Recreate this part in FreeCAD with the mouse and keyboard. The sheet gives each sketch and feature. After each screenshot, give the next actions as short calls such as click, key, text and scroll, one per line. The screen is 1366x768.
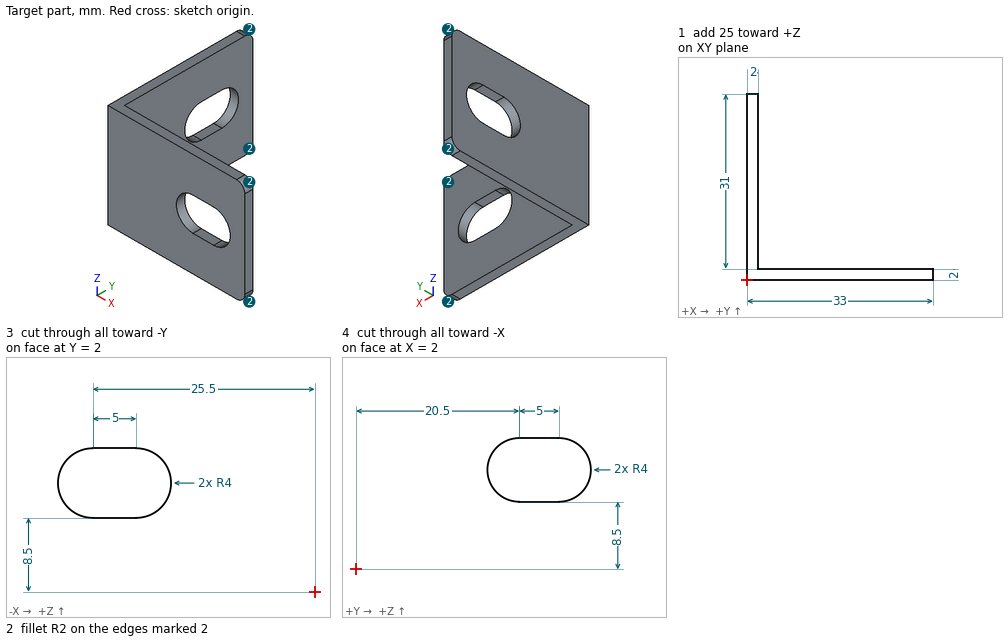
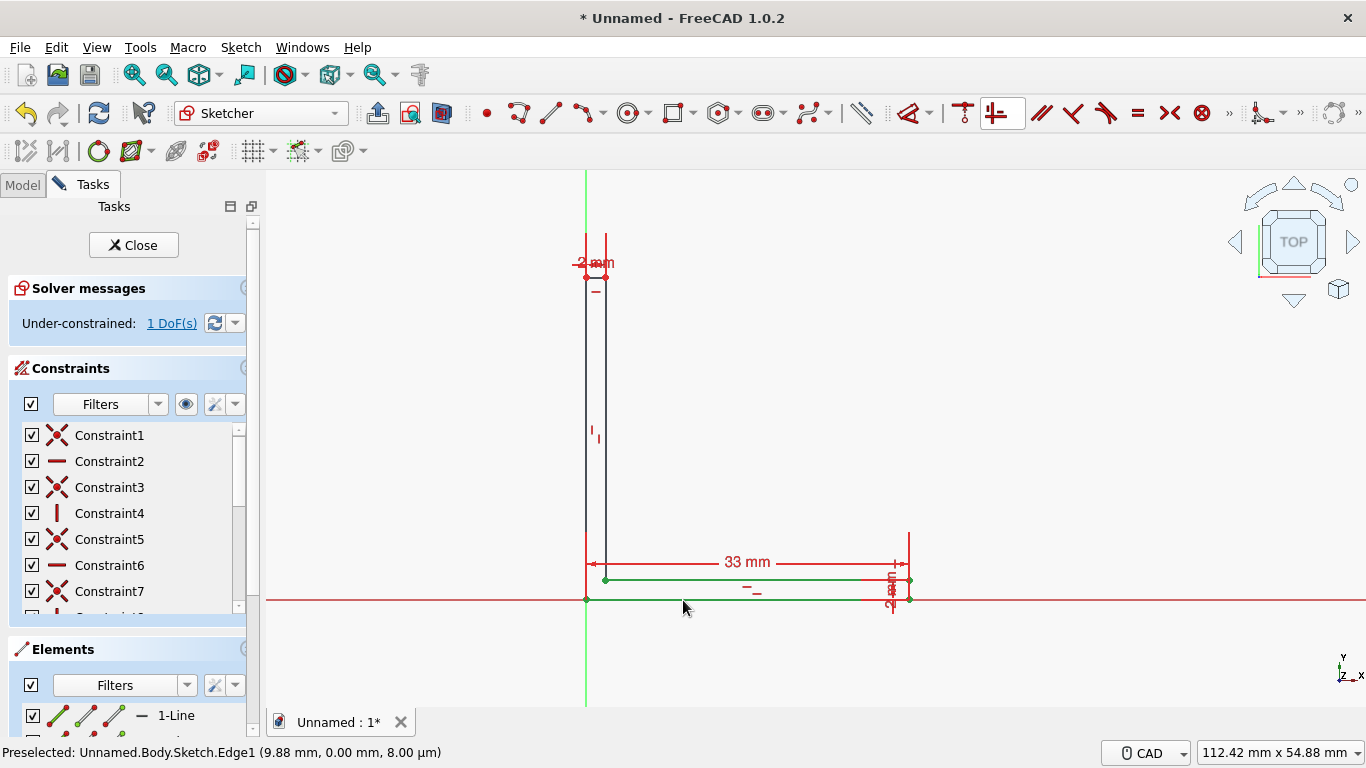
click(606, 490)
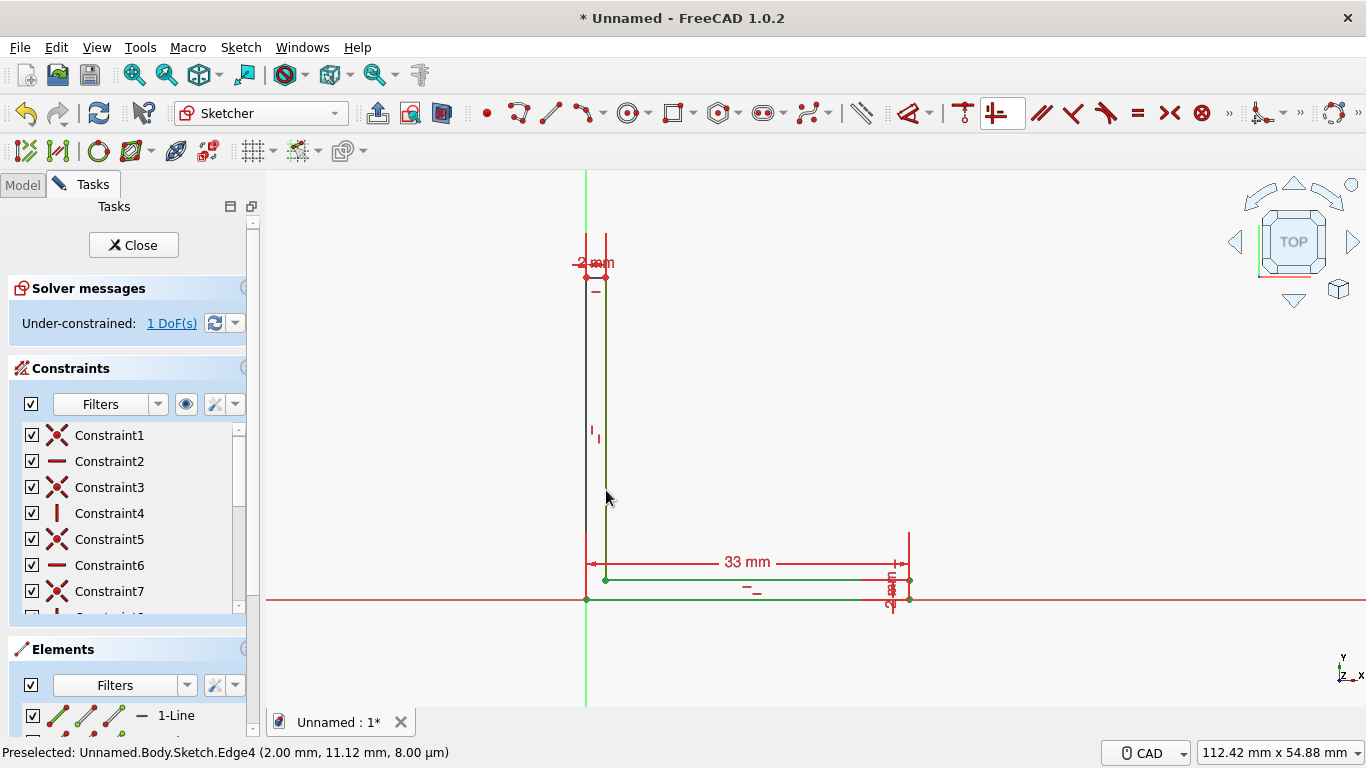
key(i)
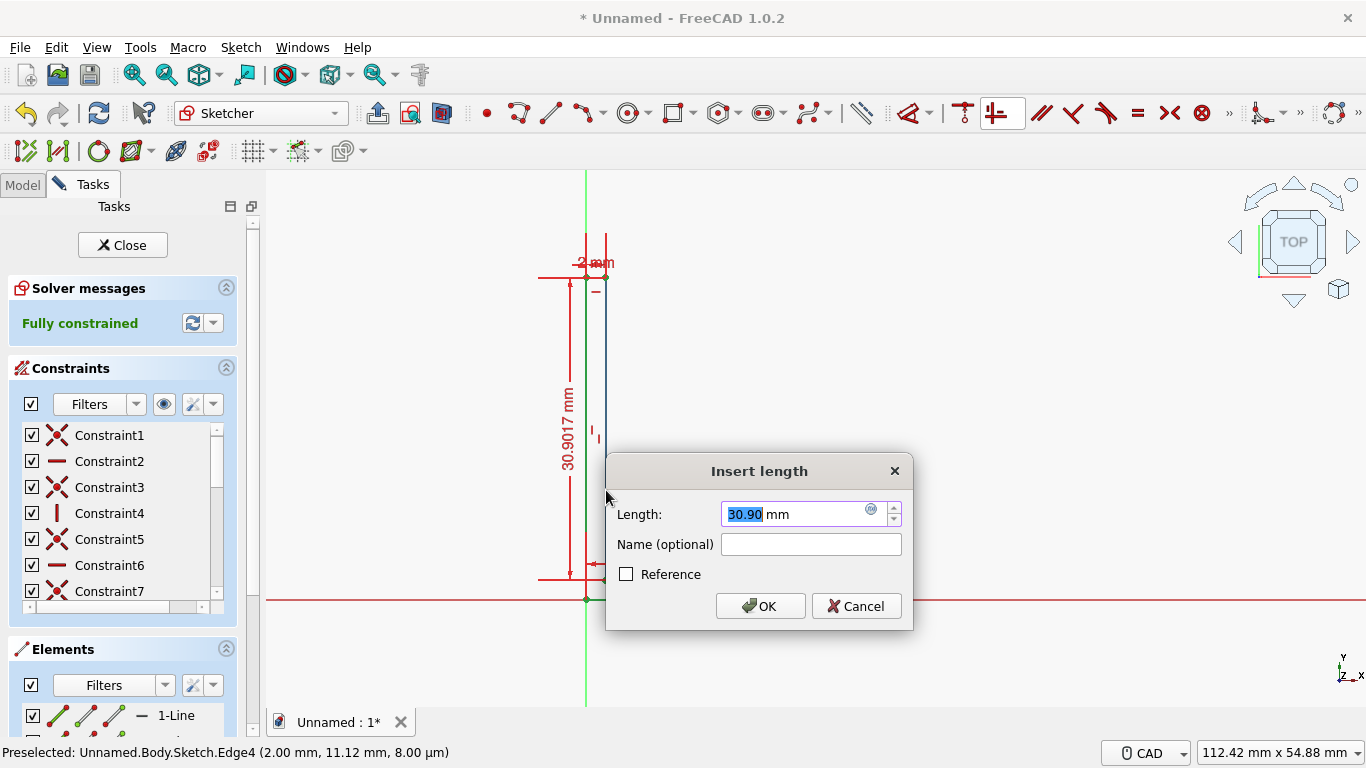
text(31)
key(Return)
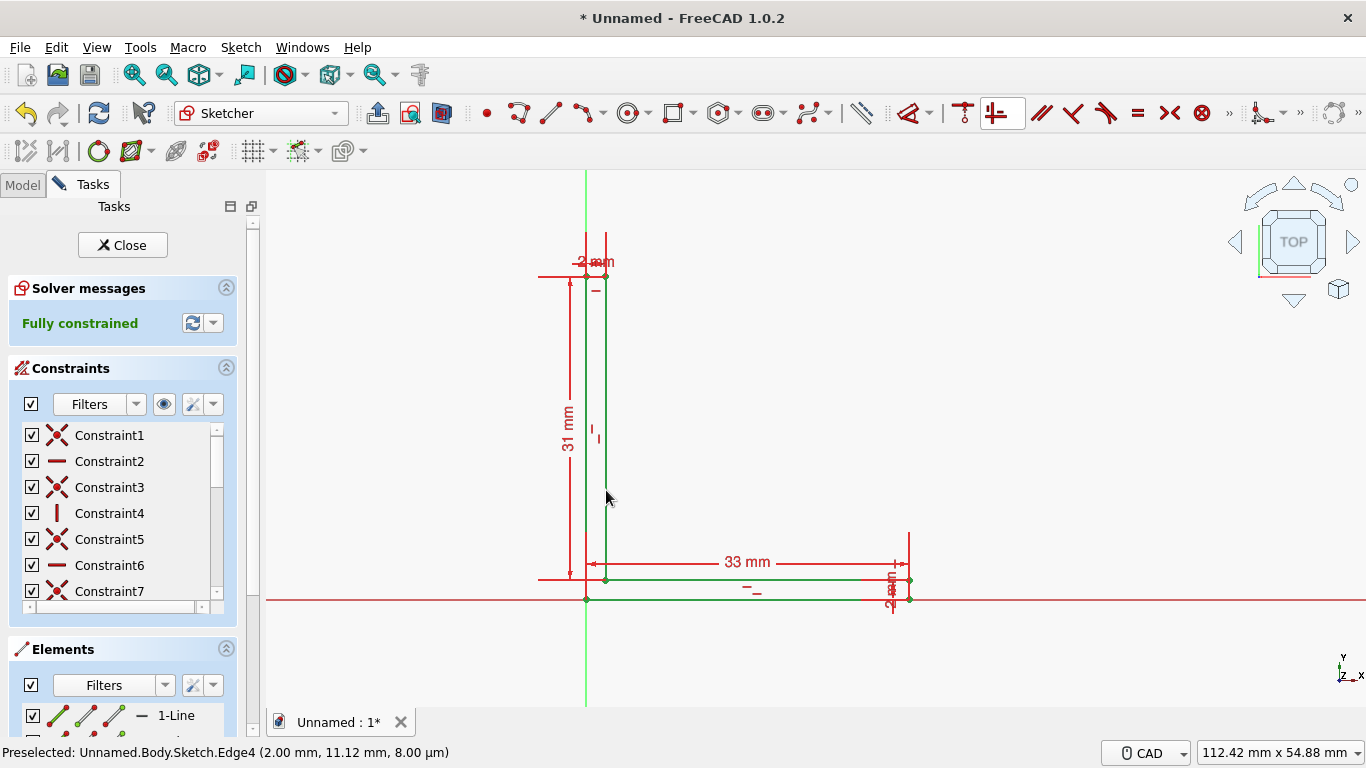
click(123, 245)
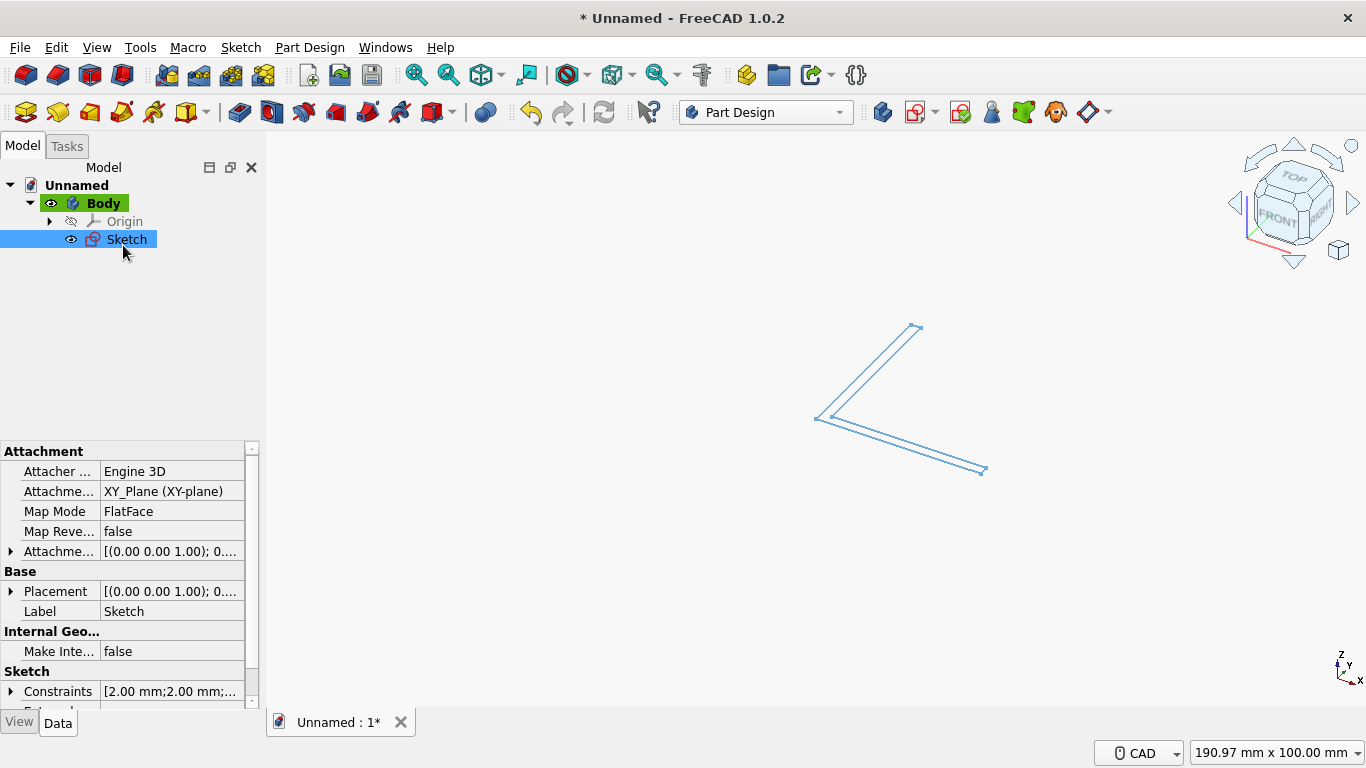
click(26, 112)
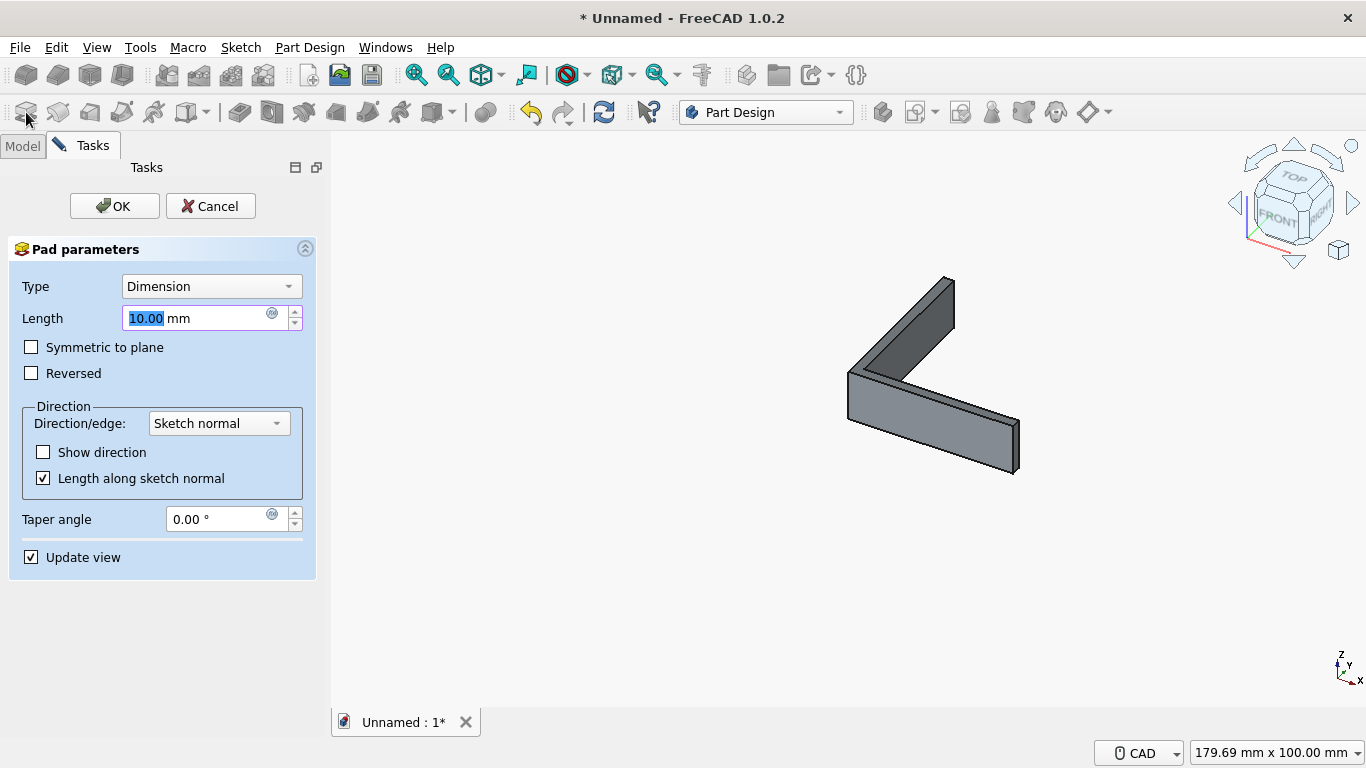
text(25)
key(Tab)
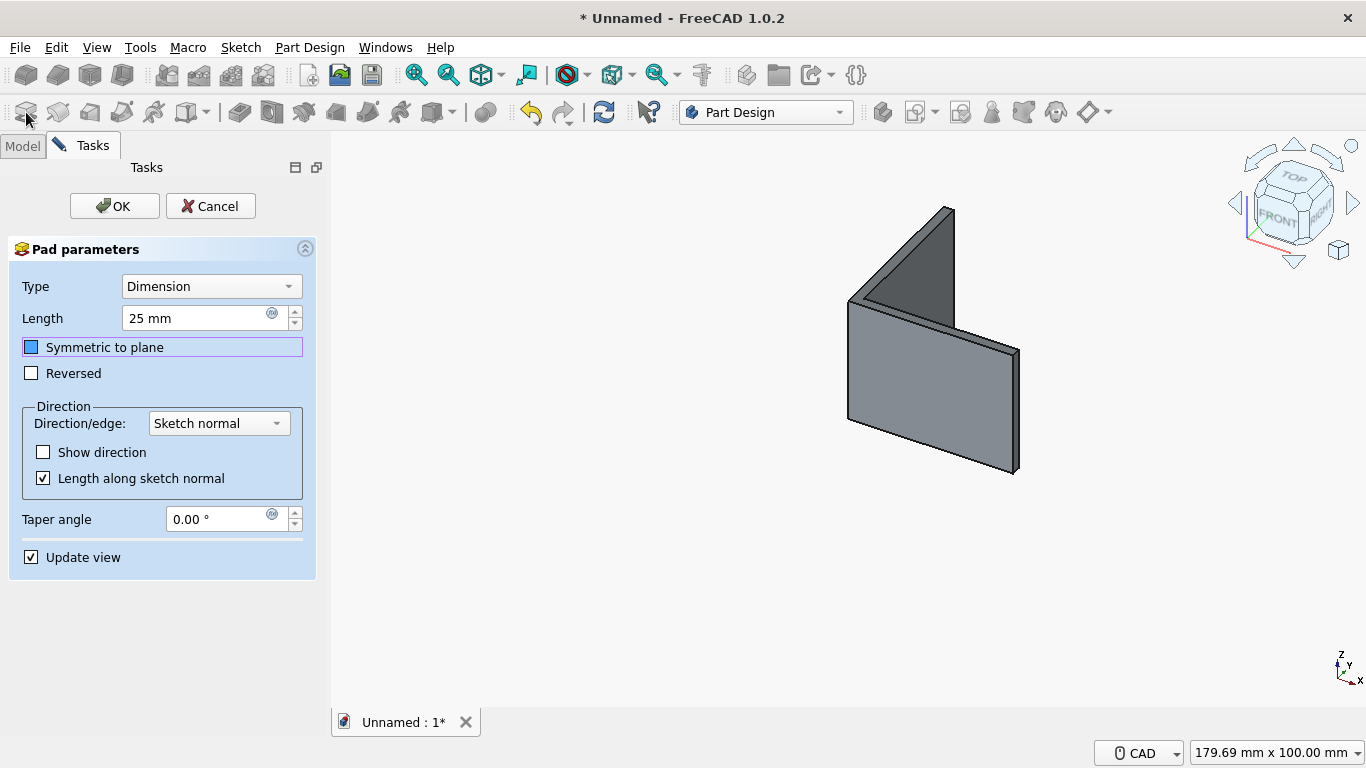
click(115, 206)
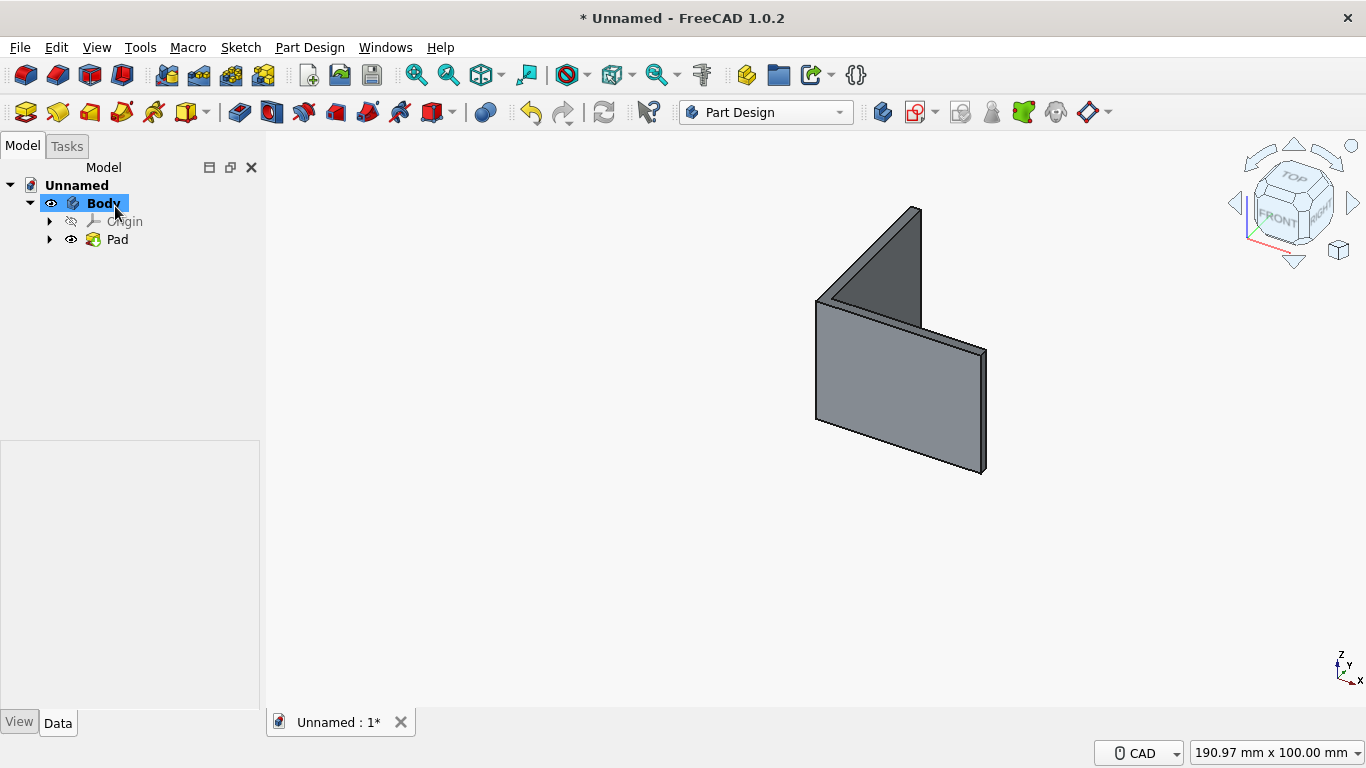
scroll(983, 352, up, 7)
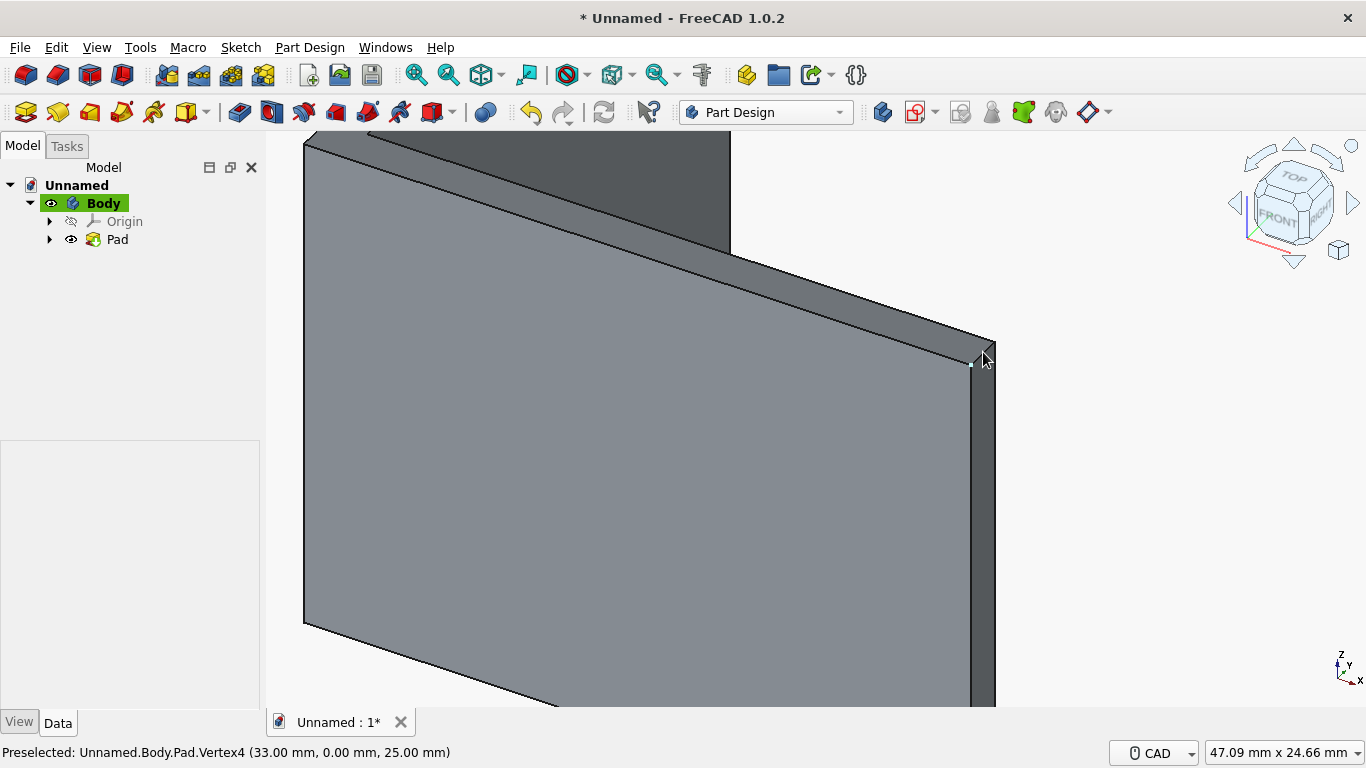
click(983, 353)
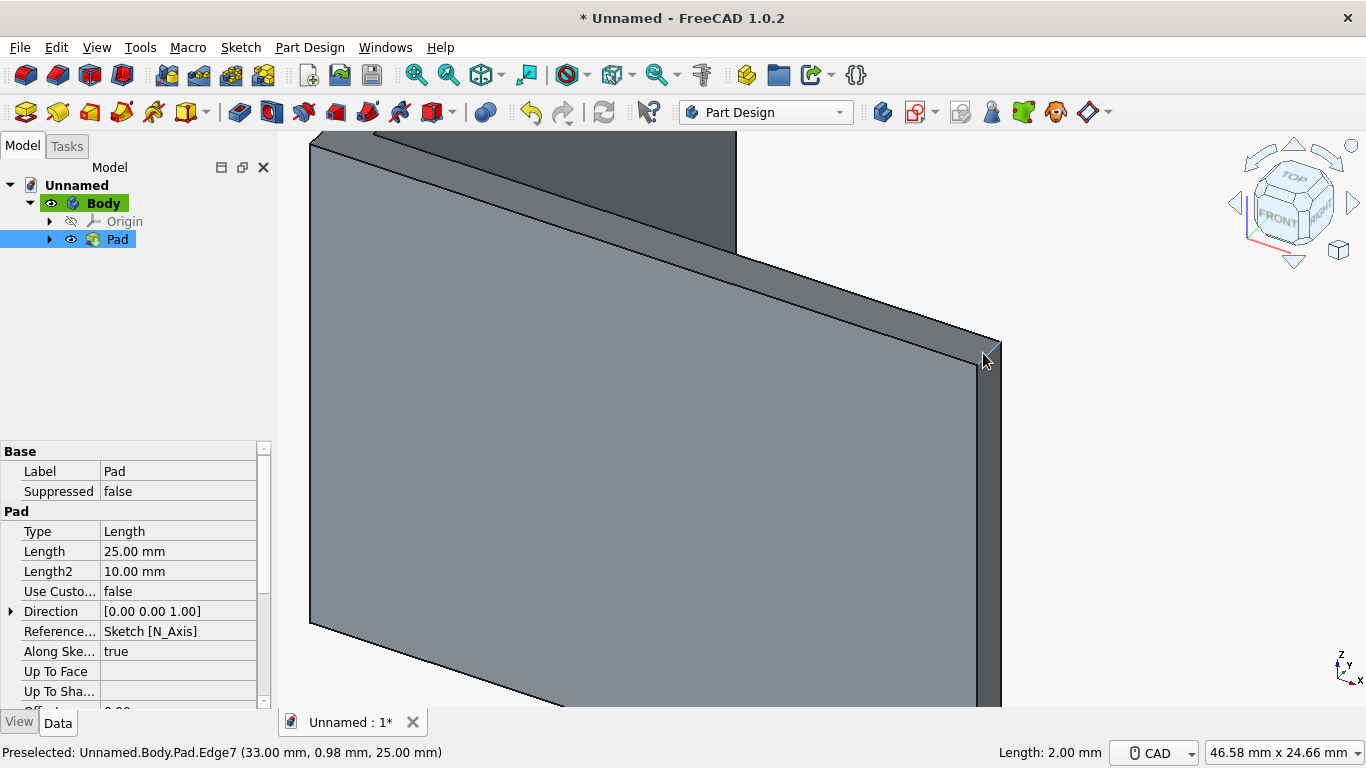
click(418, 76)